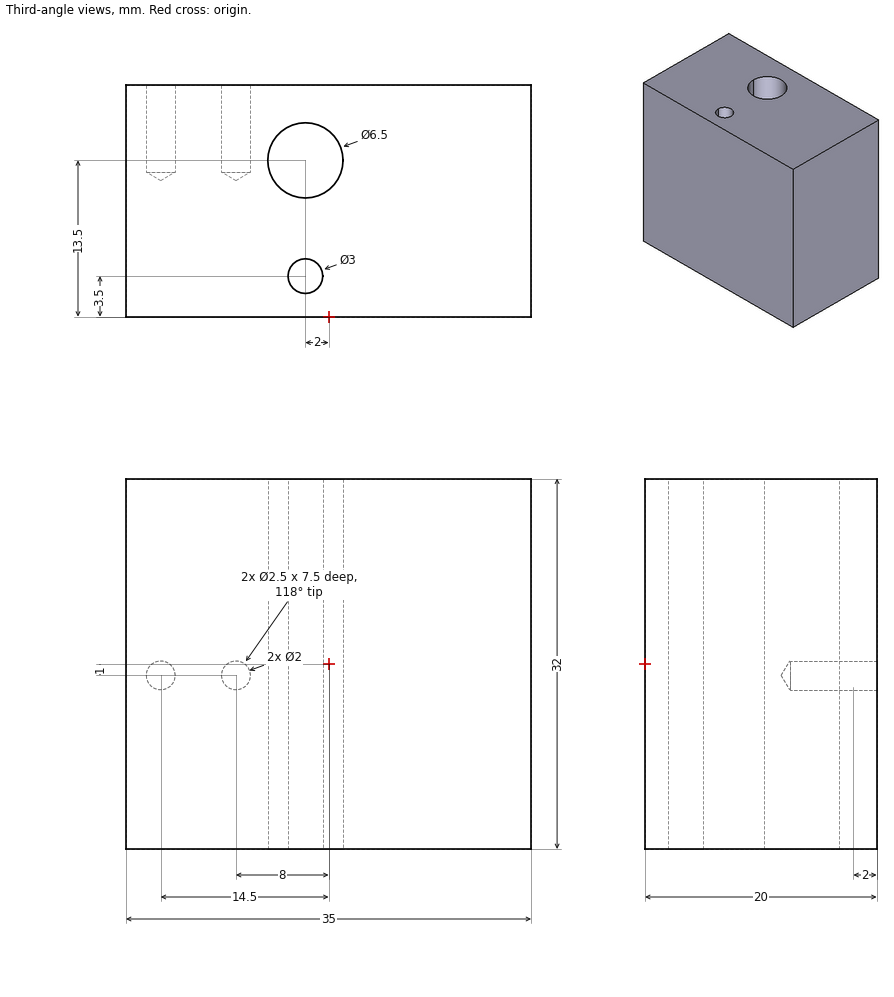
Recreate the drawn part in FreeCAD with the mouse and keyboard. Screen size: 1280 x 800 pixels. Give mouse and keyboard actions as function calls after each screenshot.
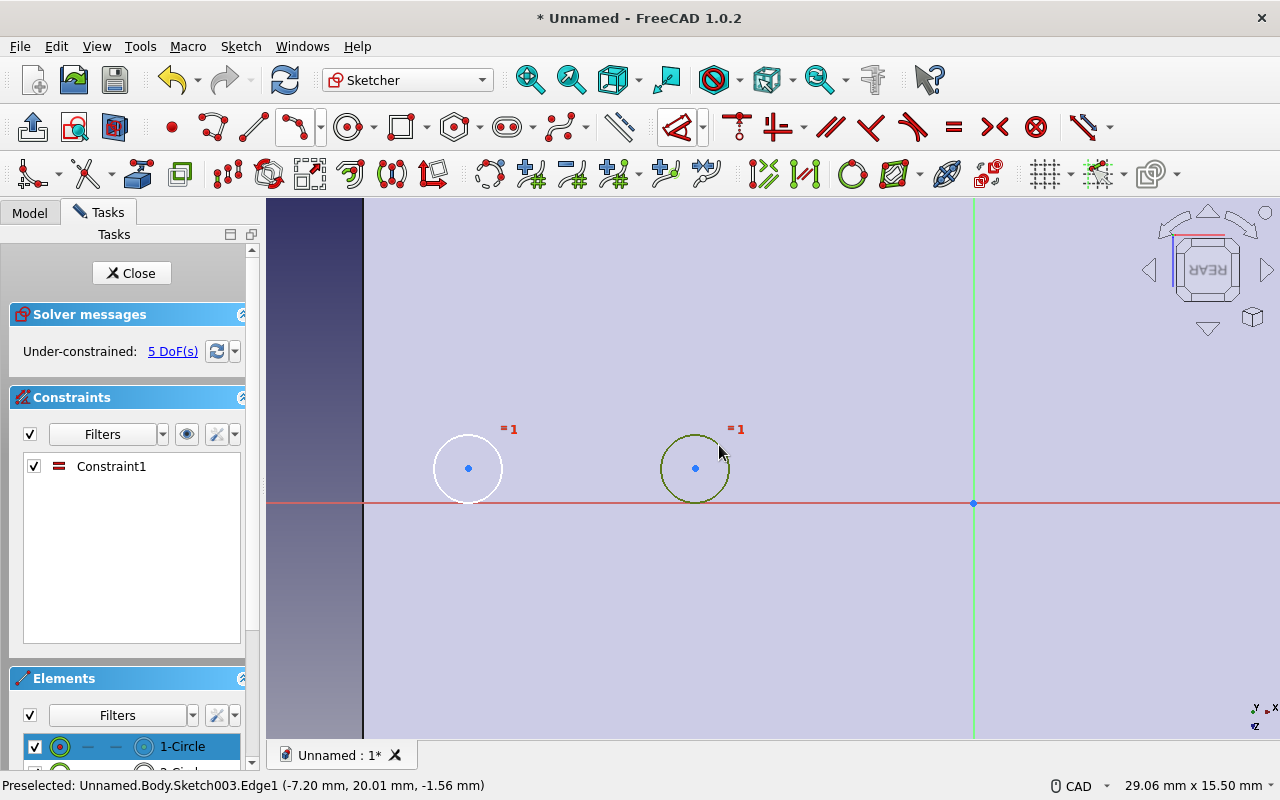
click(702, 128)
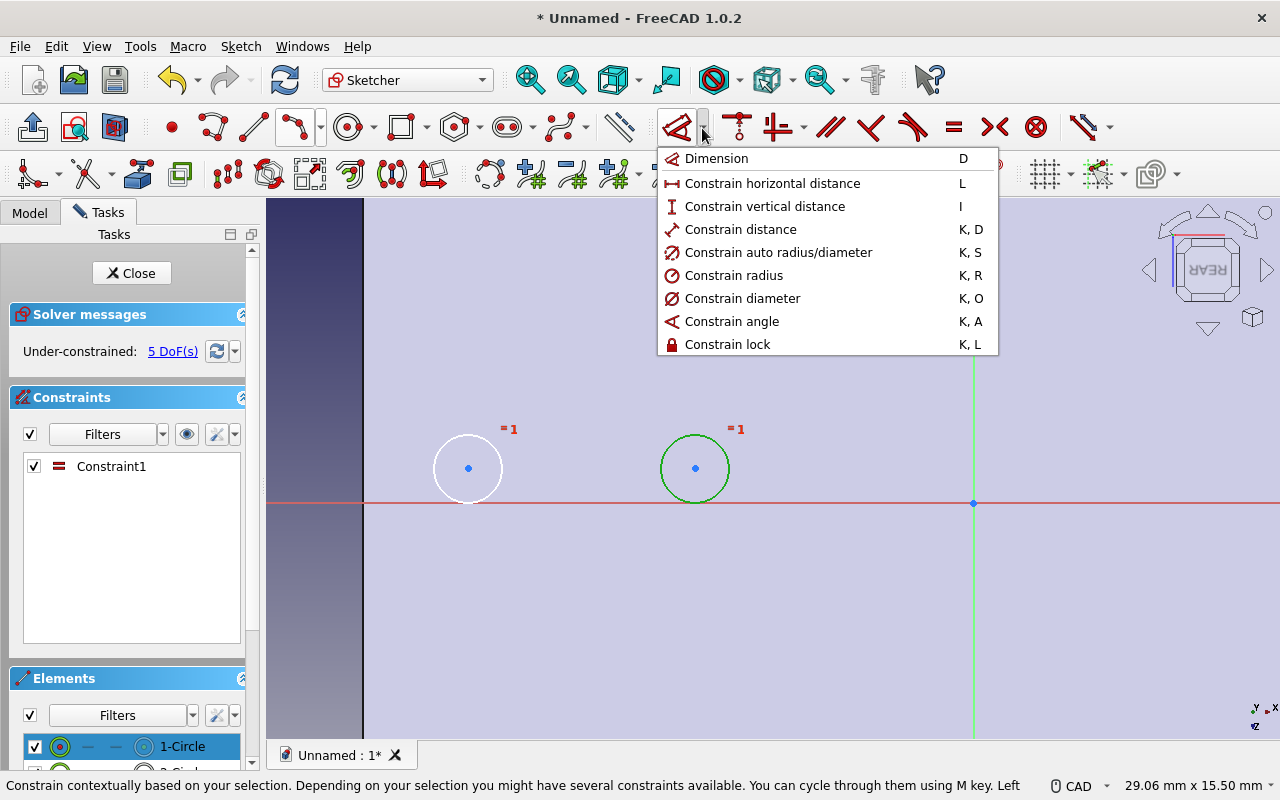
click(828, 298)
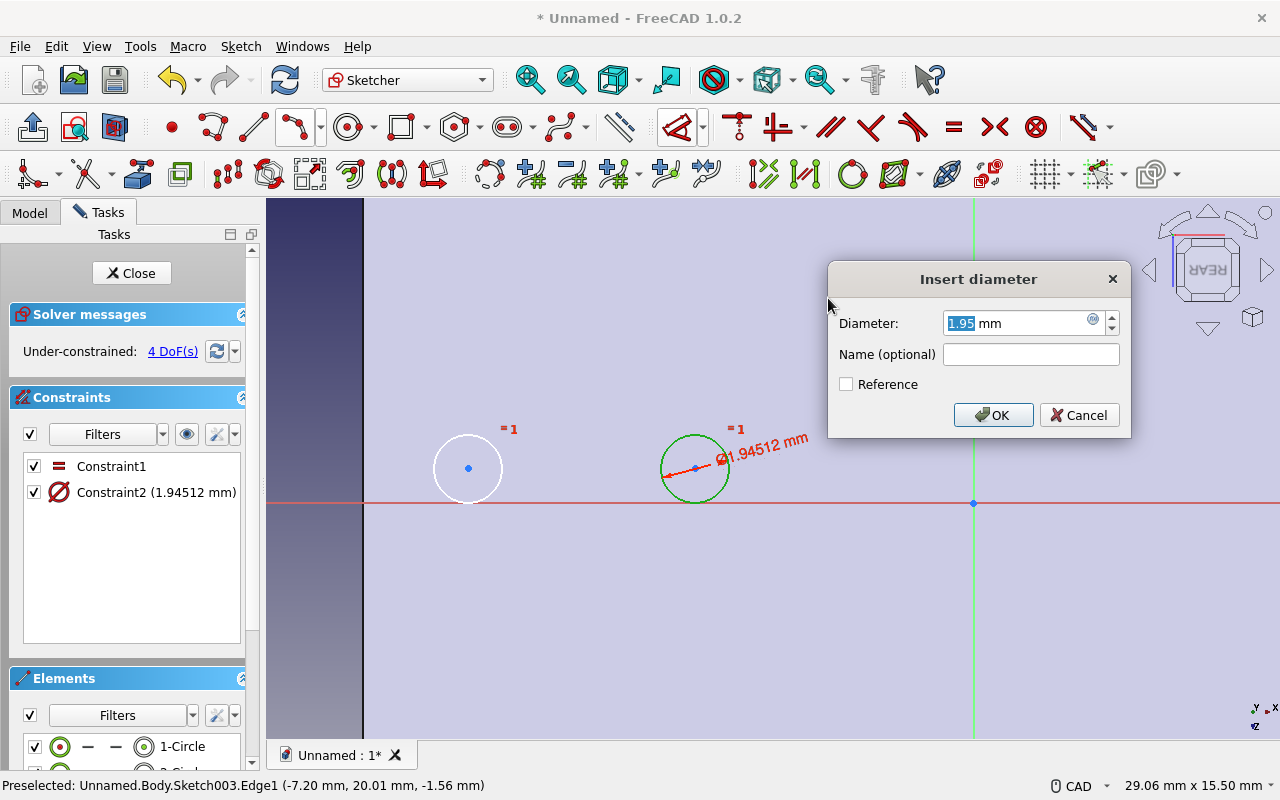
text(2)
key(Return)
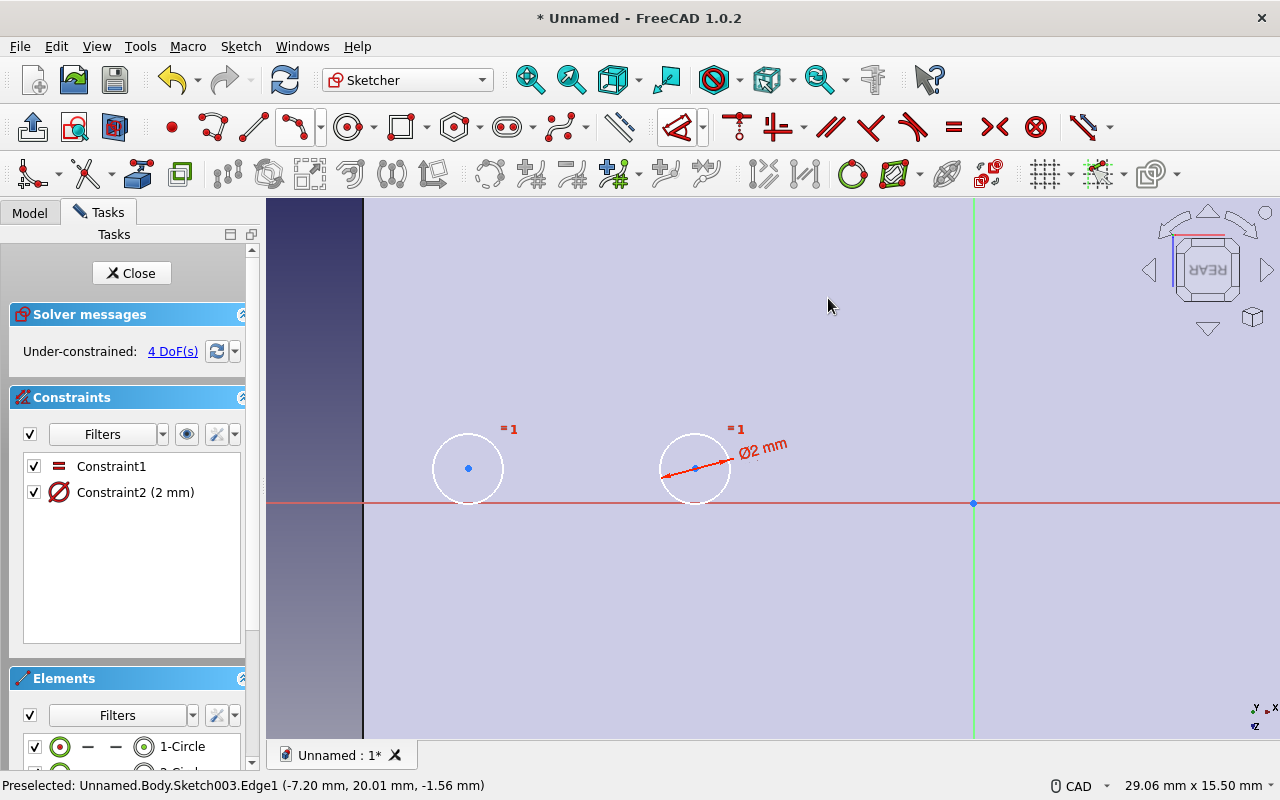
click(695, 469)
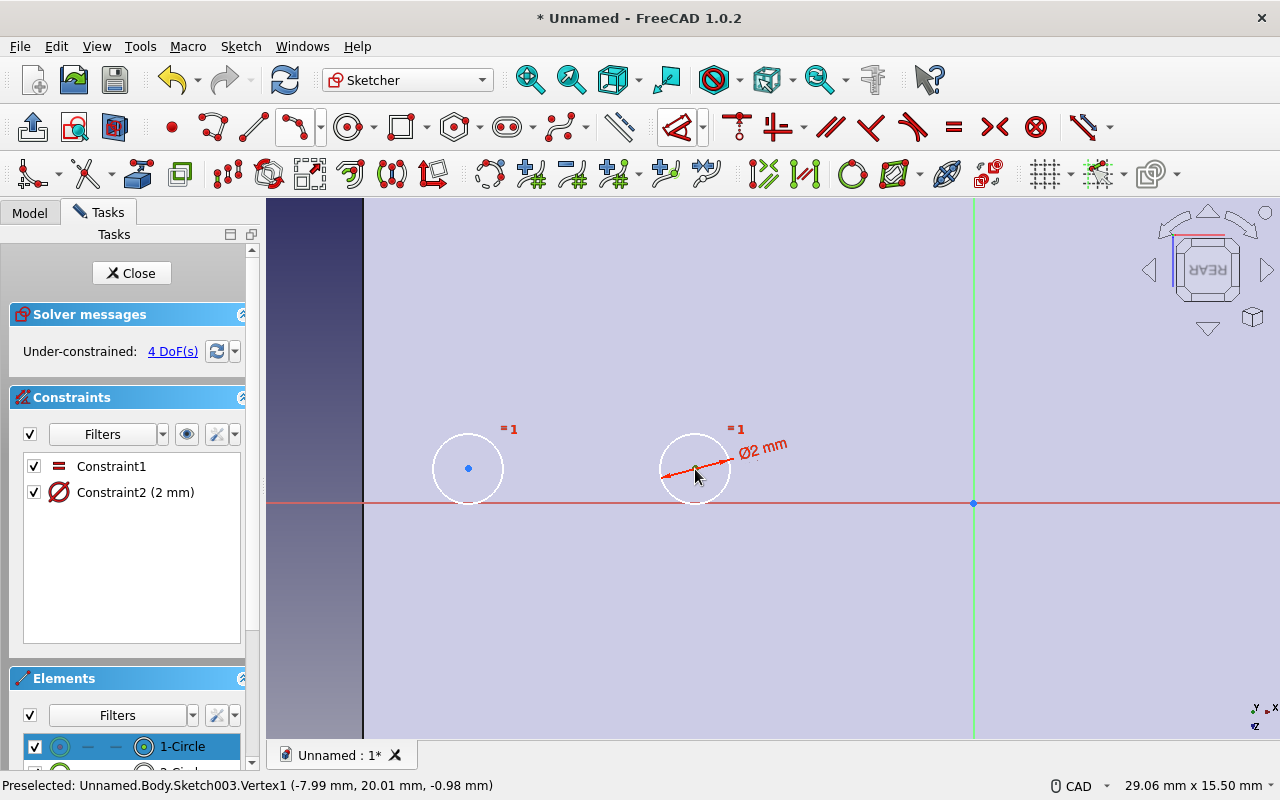
key(l)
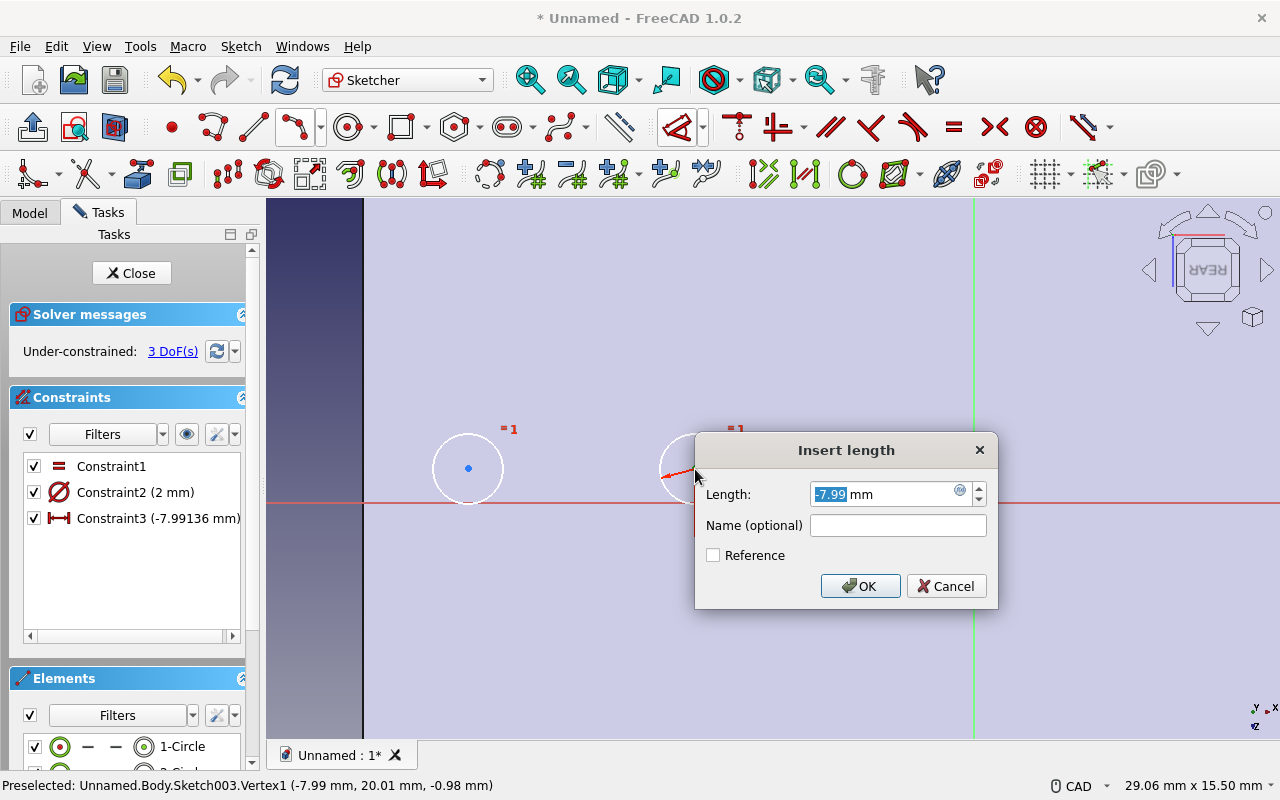
text(-8)
key(Return)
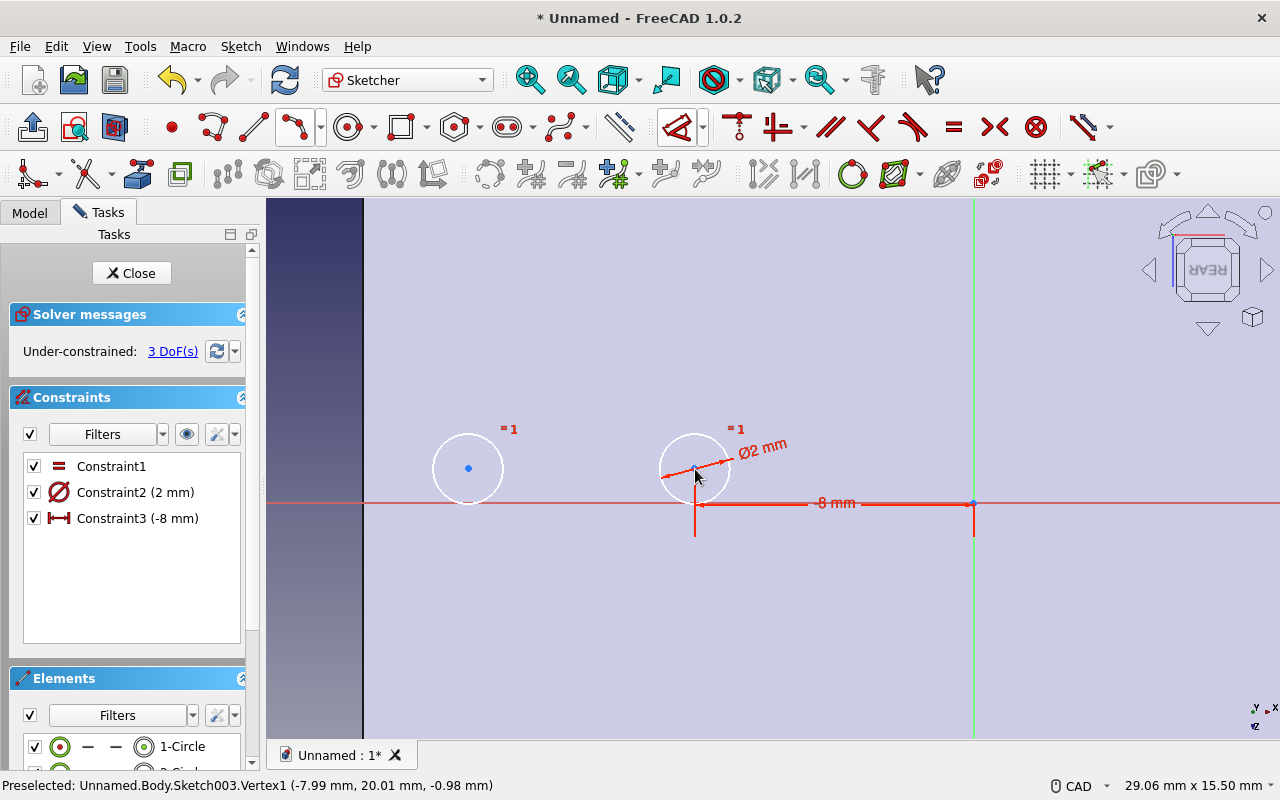
click(695, 469)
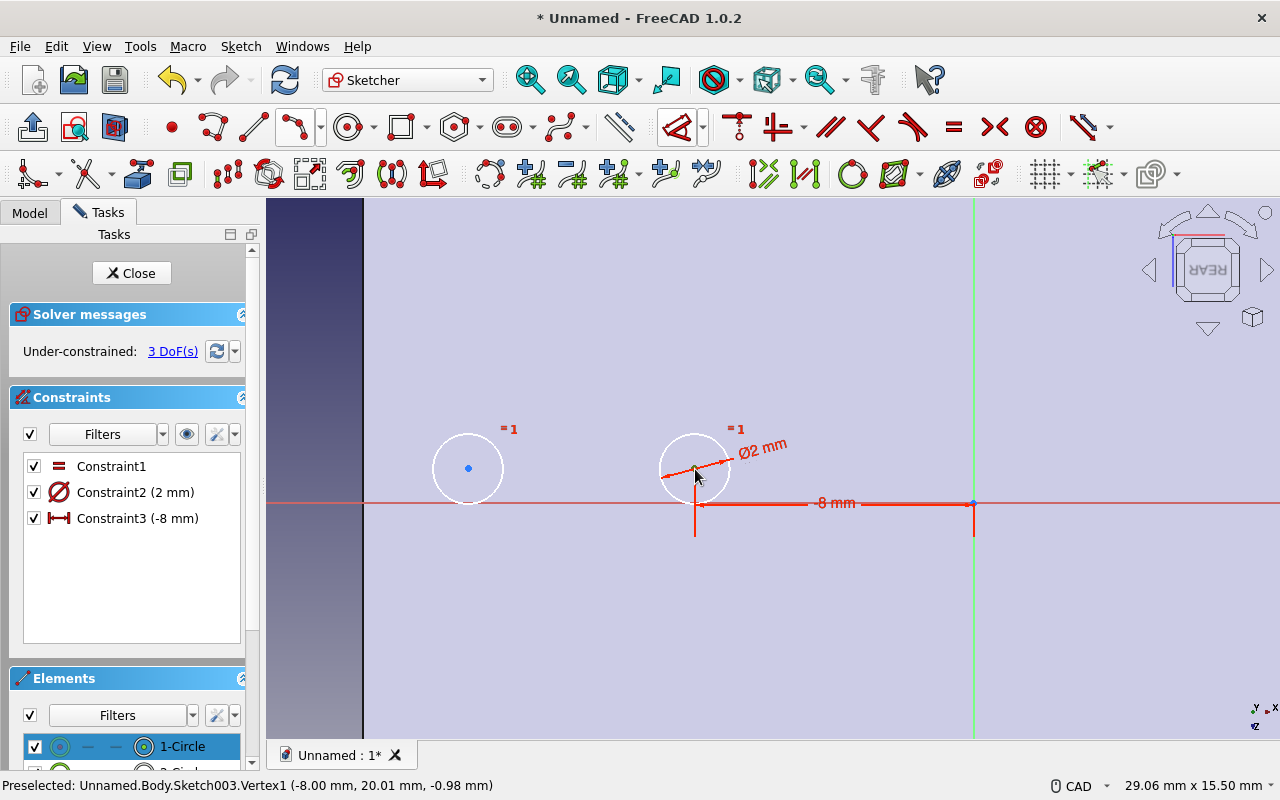
key(i)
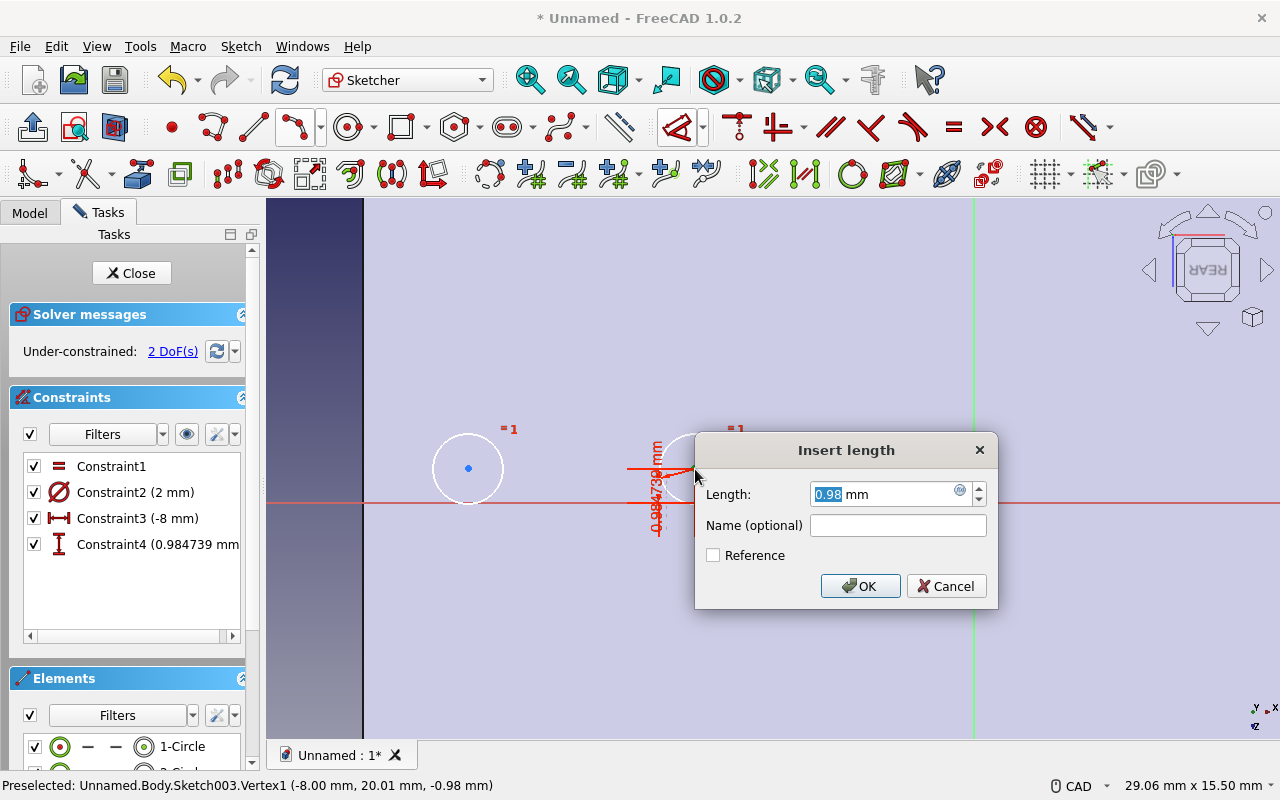
text(1)
key(Return)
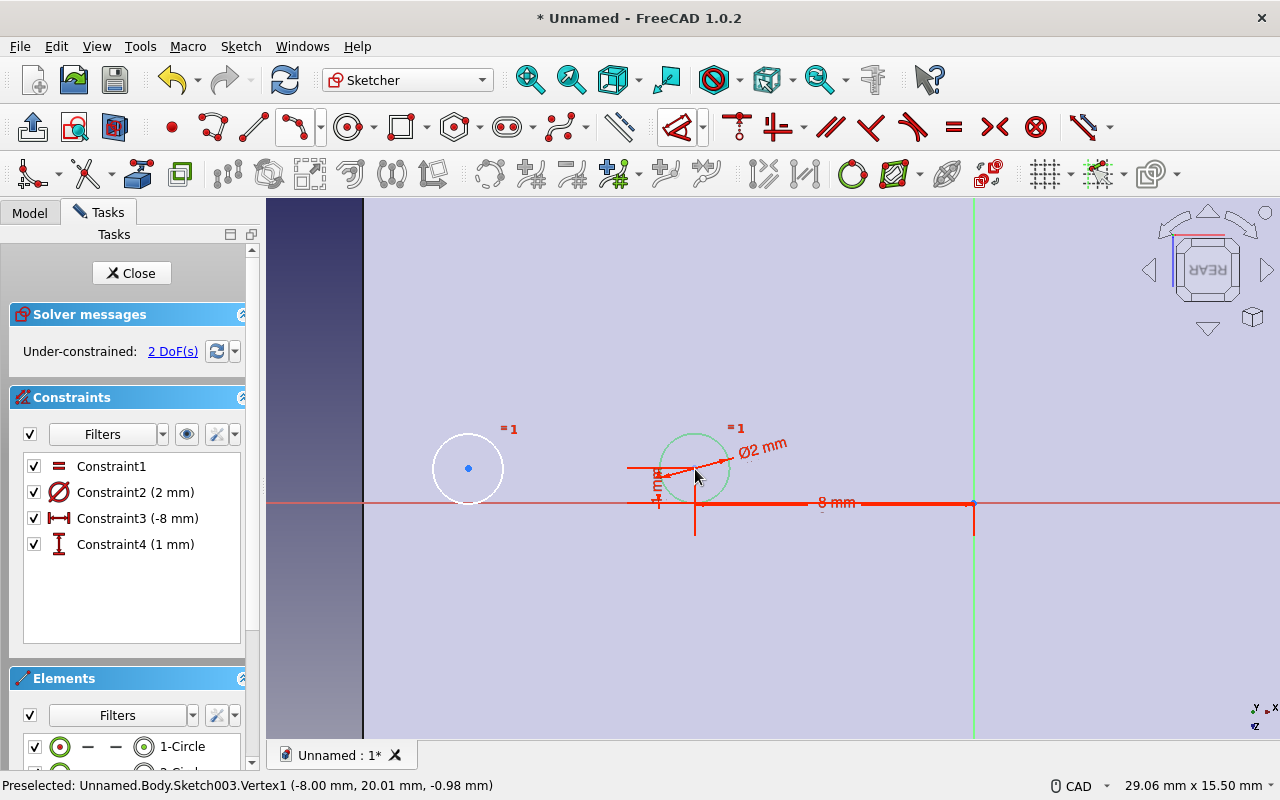
click(468, 469)